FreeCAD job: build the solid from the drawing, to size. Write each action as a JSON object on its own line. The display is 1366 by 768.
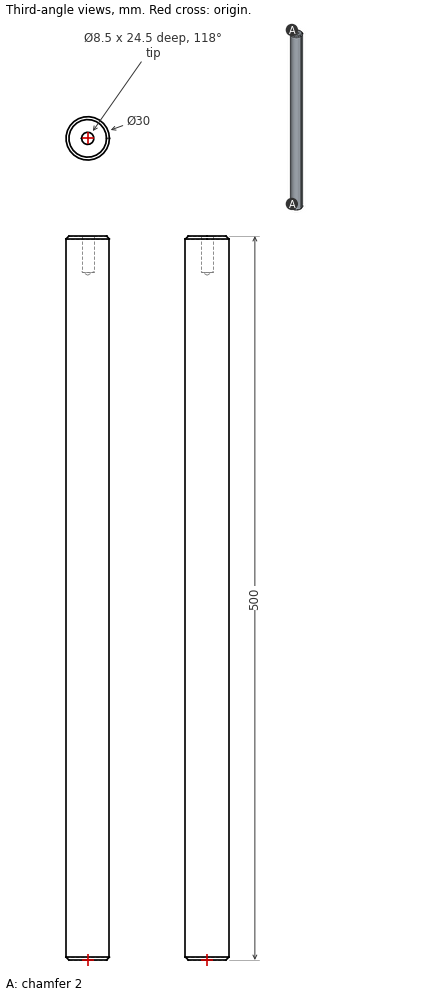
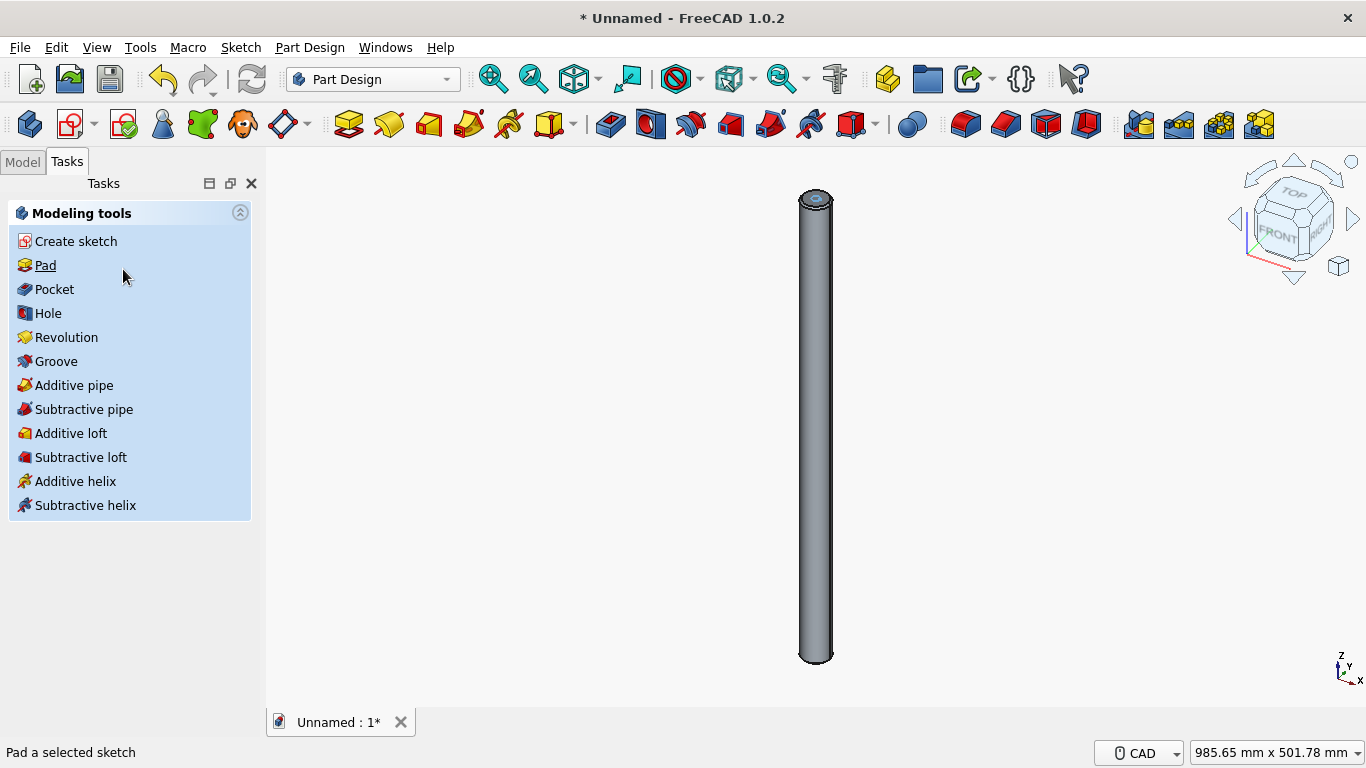
{"action": "left_click", "coordinate": [652, 124]}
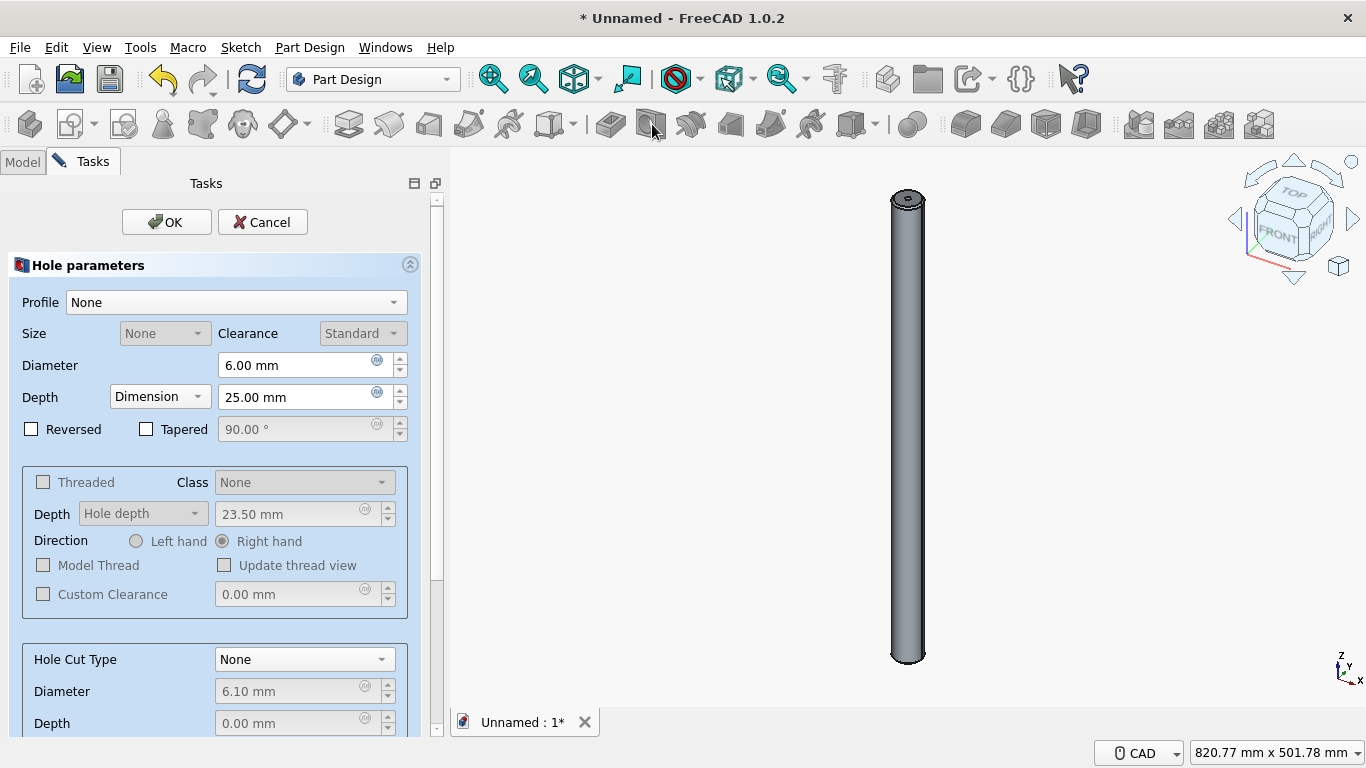
{"action": "triple_click", "coordinate": [305, 365]}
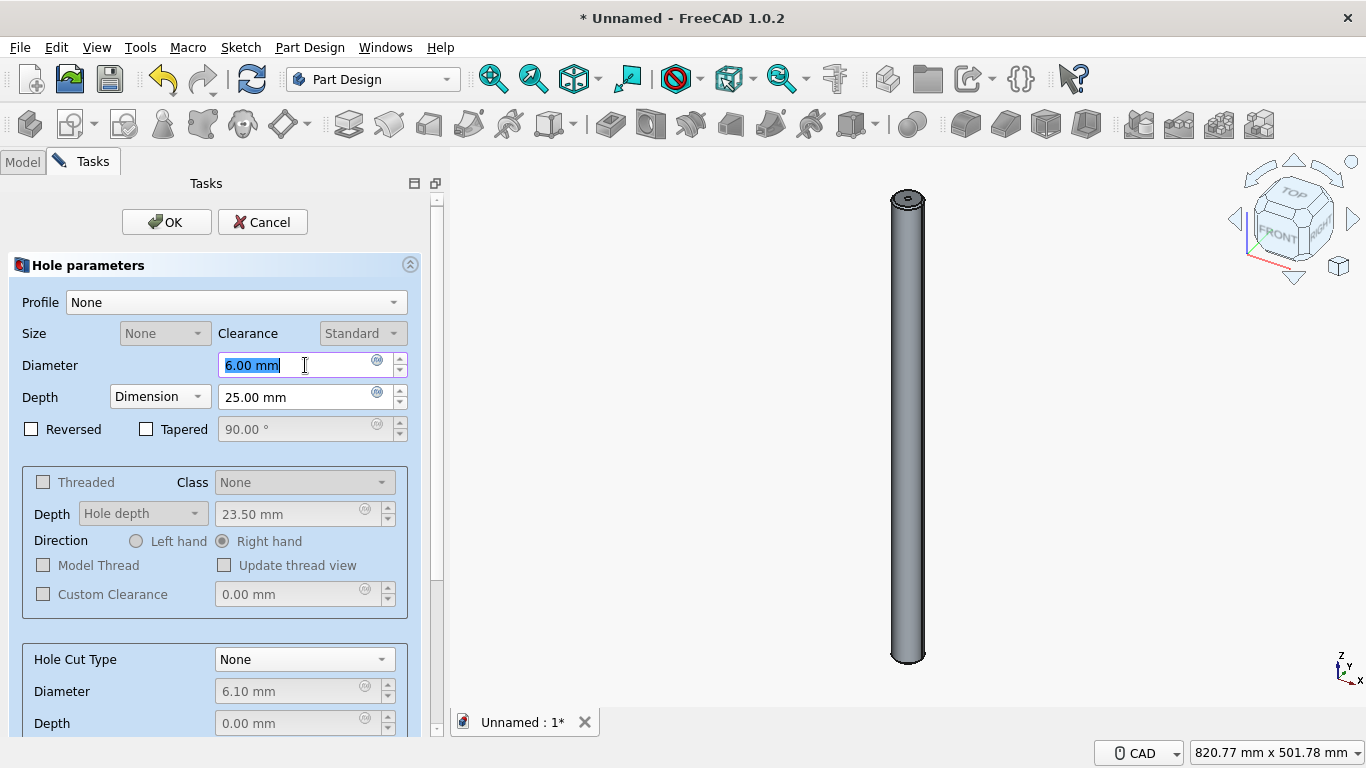
{"action": "type", "text": "8.5"}
{"action": "key", "text": "Tab"}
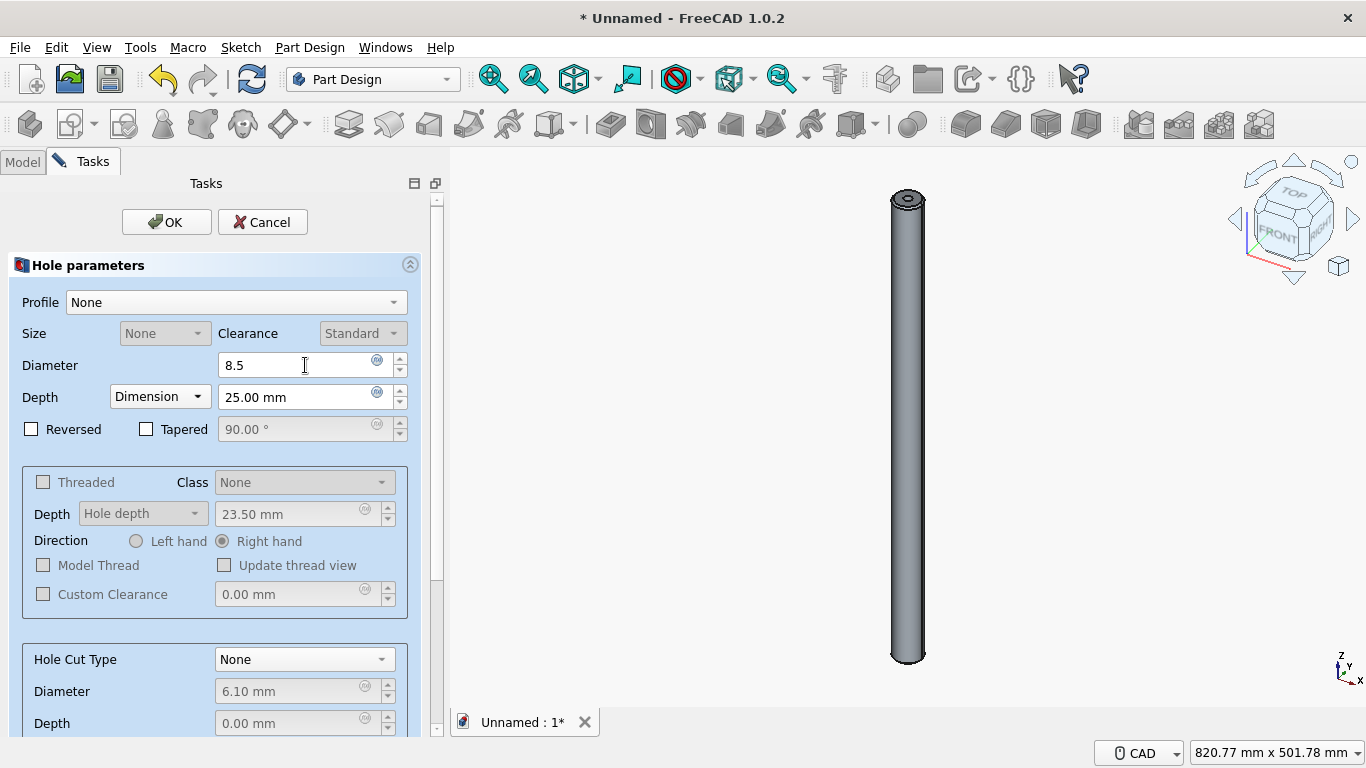
{"action": "triple_click", "coordinate": [305, 397]}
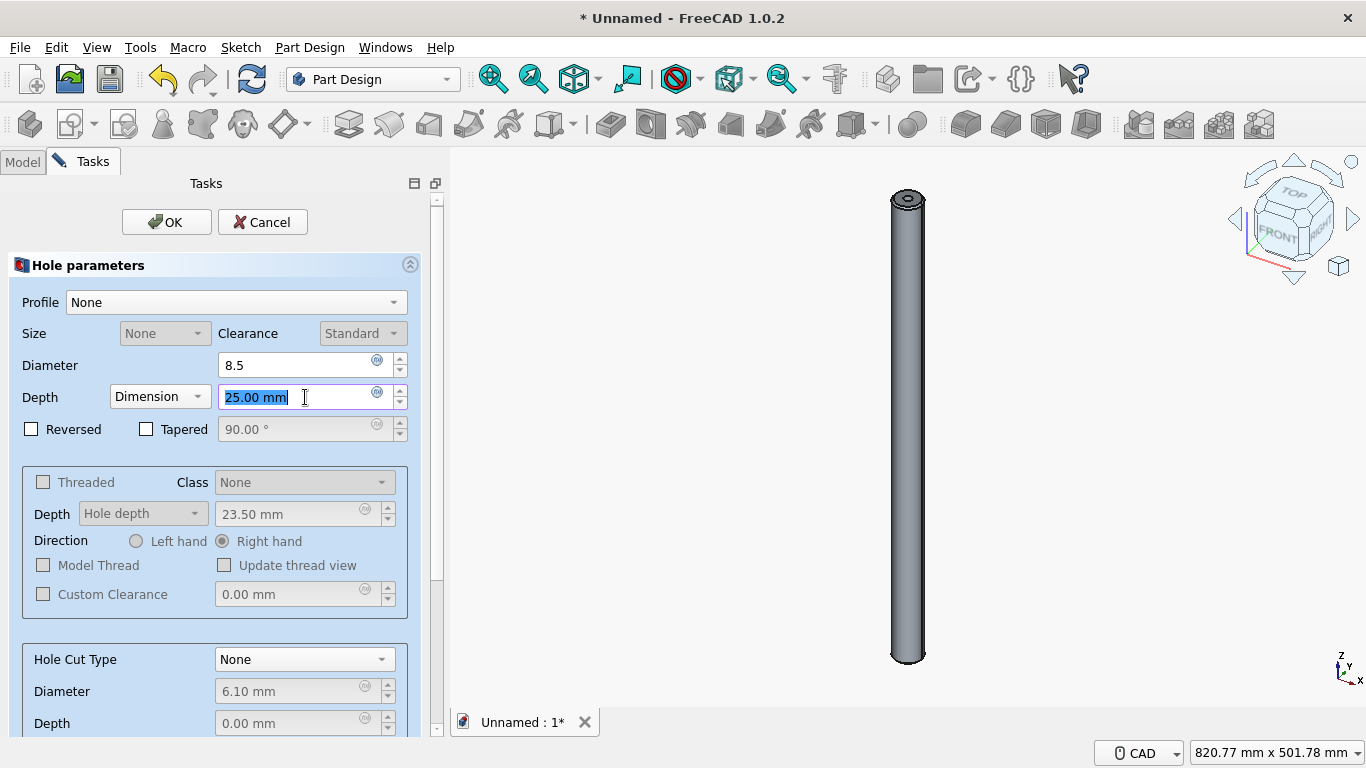
{"action": "type", "text": "24.5"}
{"action": "key", "text": "Tab"}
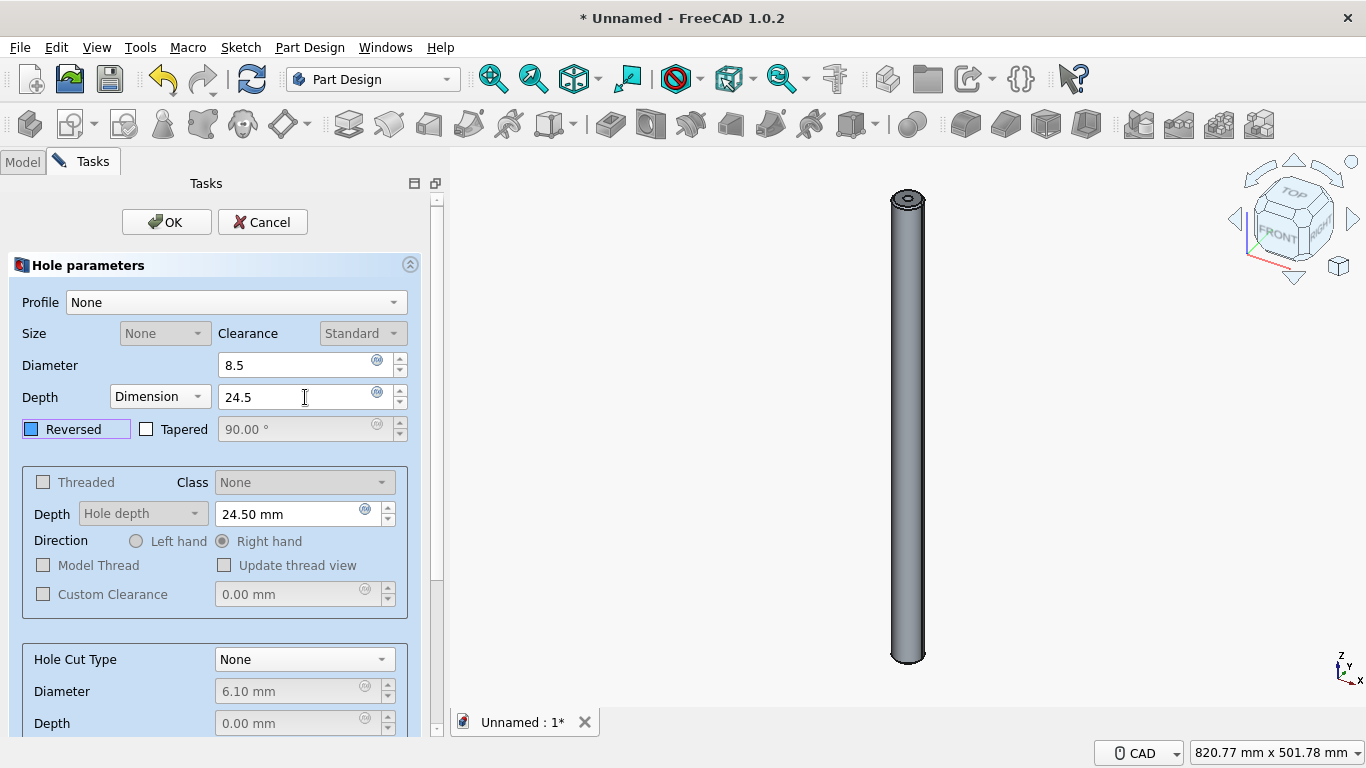
{"action": "left_click", "coordinate": [167, 222]}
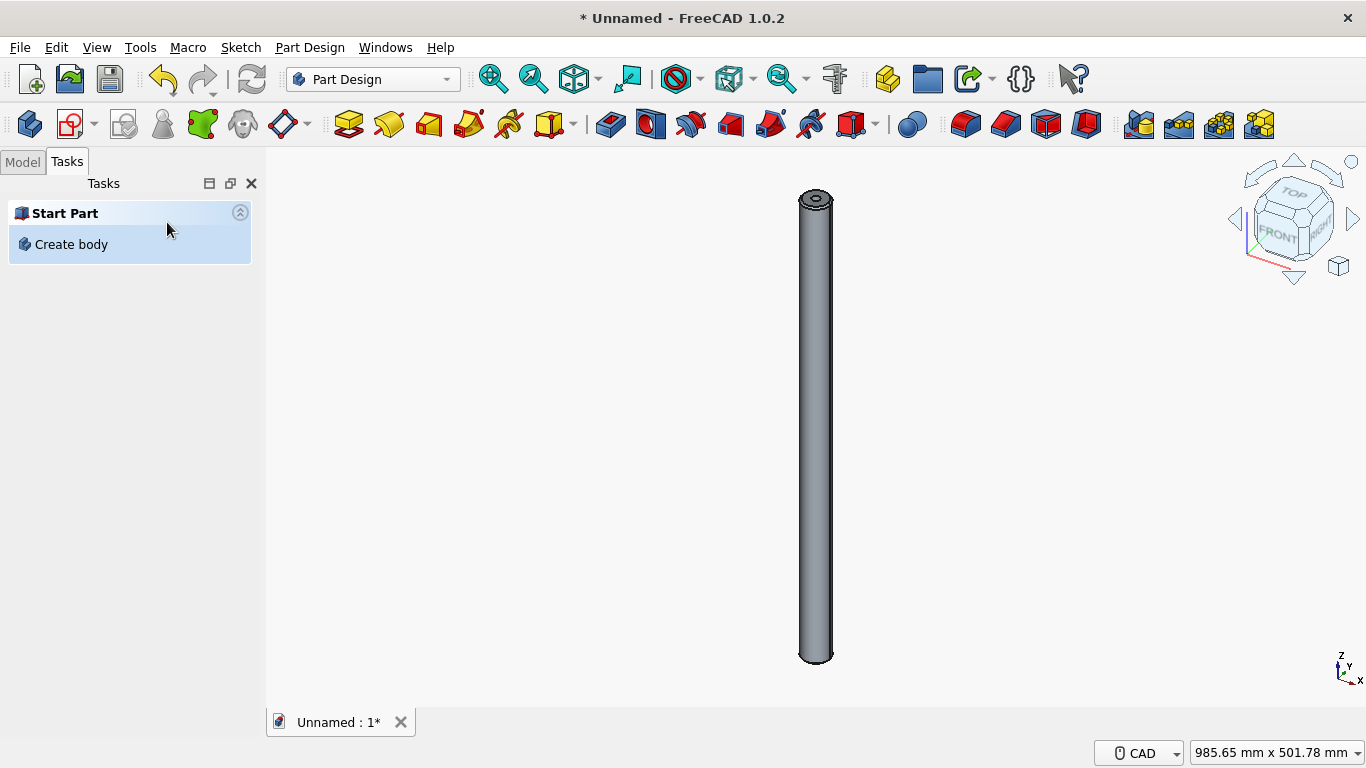
{"action": "key", "text": "0"}